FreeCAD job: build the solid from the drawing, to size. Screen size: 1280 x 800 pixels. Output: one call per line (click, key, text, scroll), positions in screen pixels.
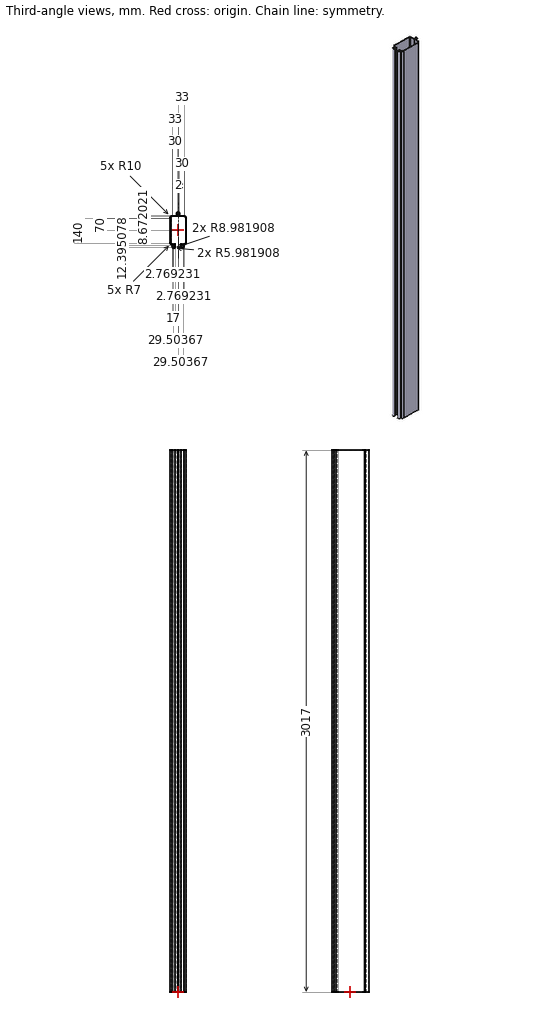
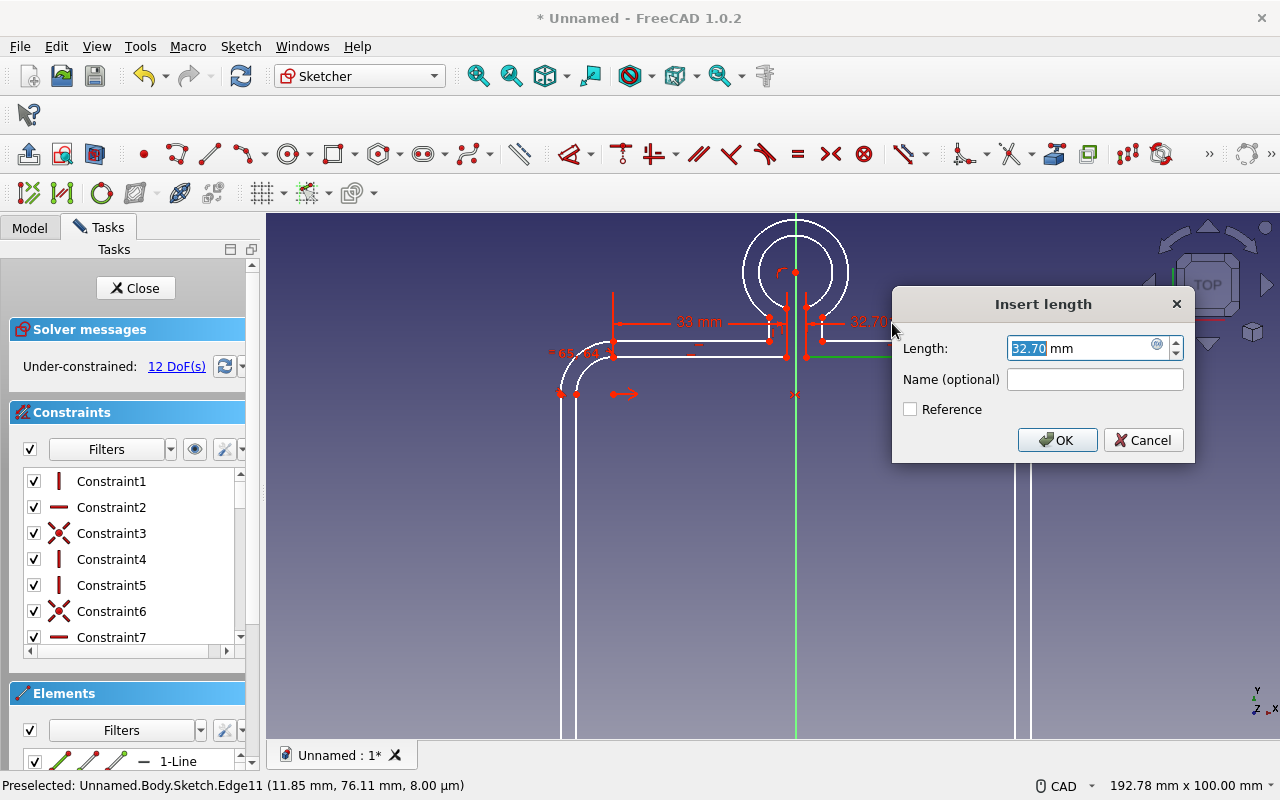
text(33)
key(Return)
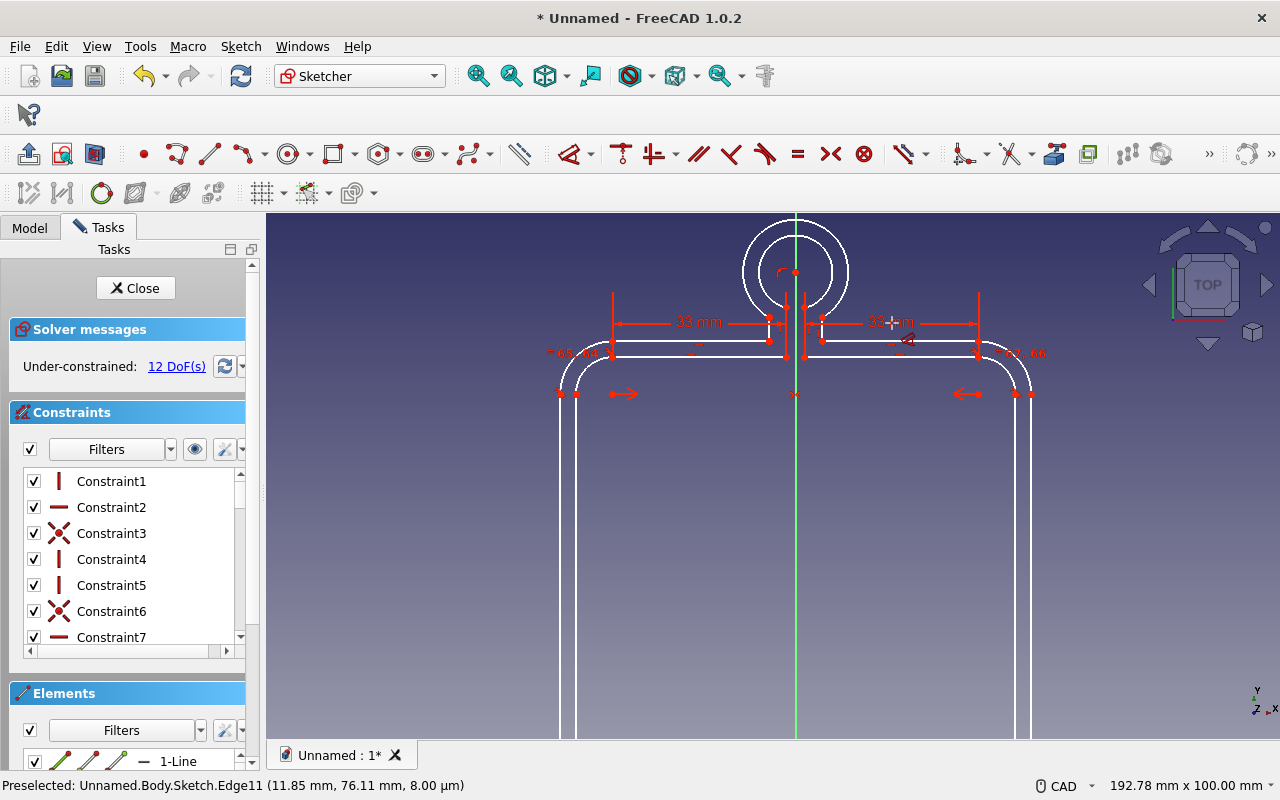
click(932, 341)
click(901, 375)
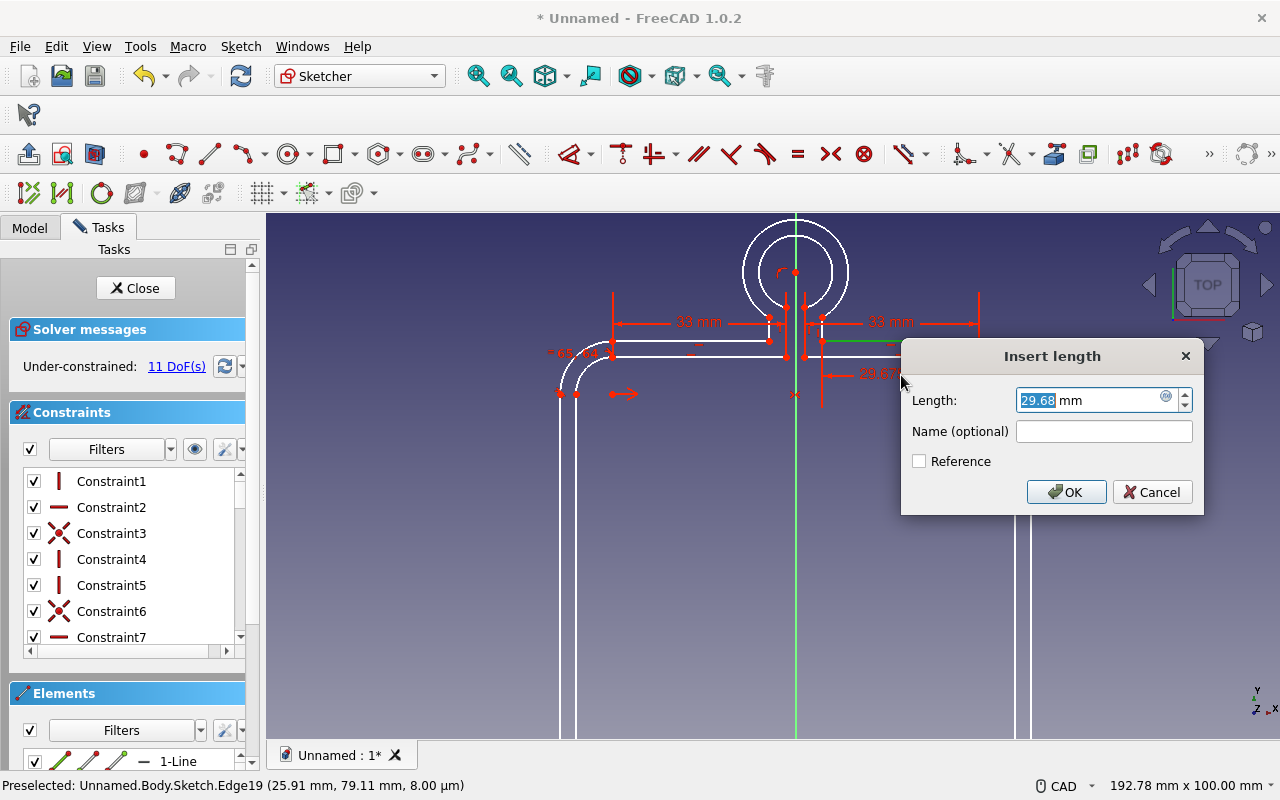
text(30)
key(Return)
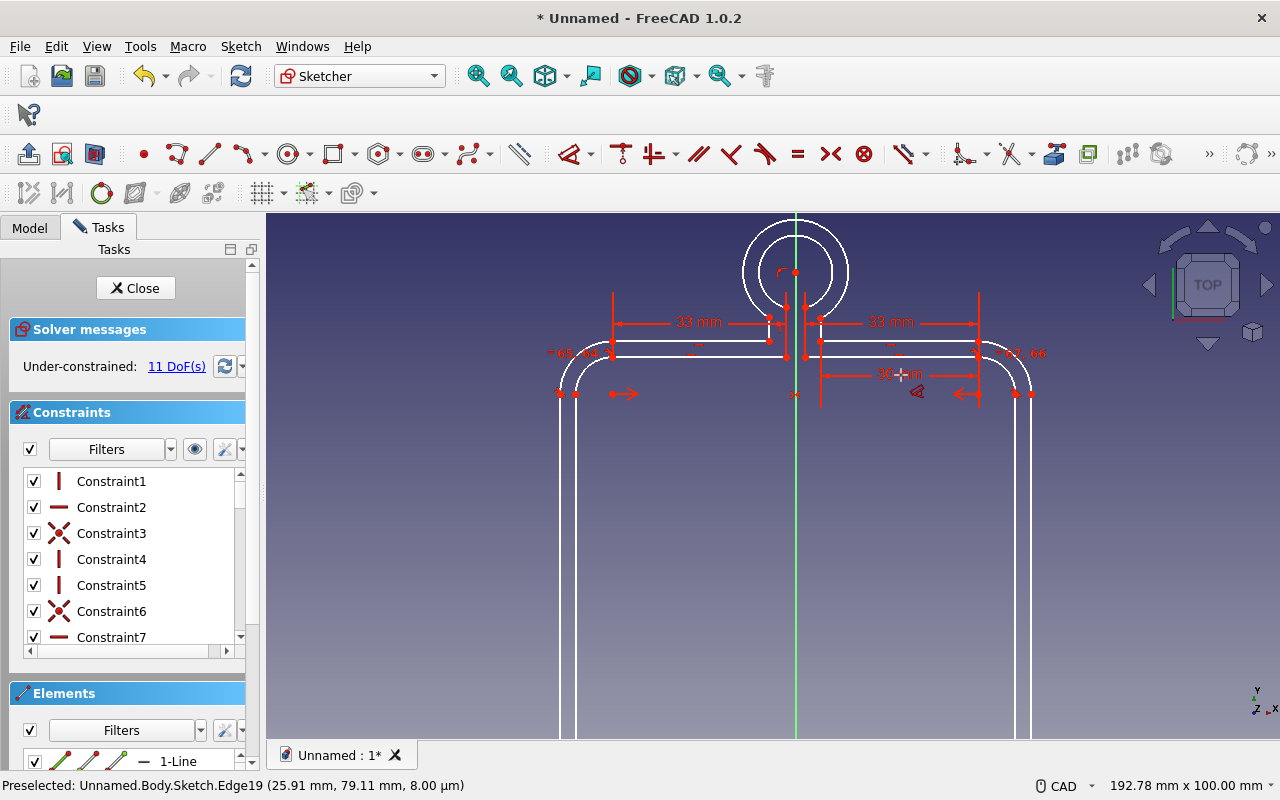
click(722, 341)
click(691, 375)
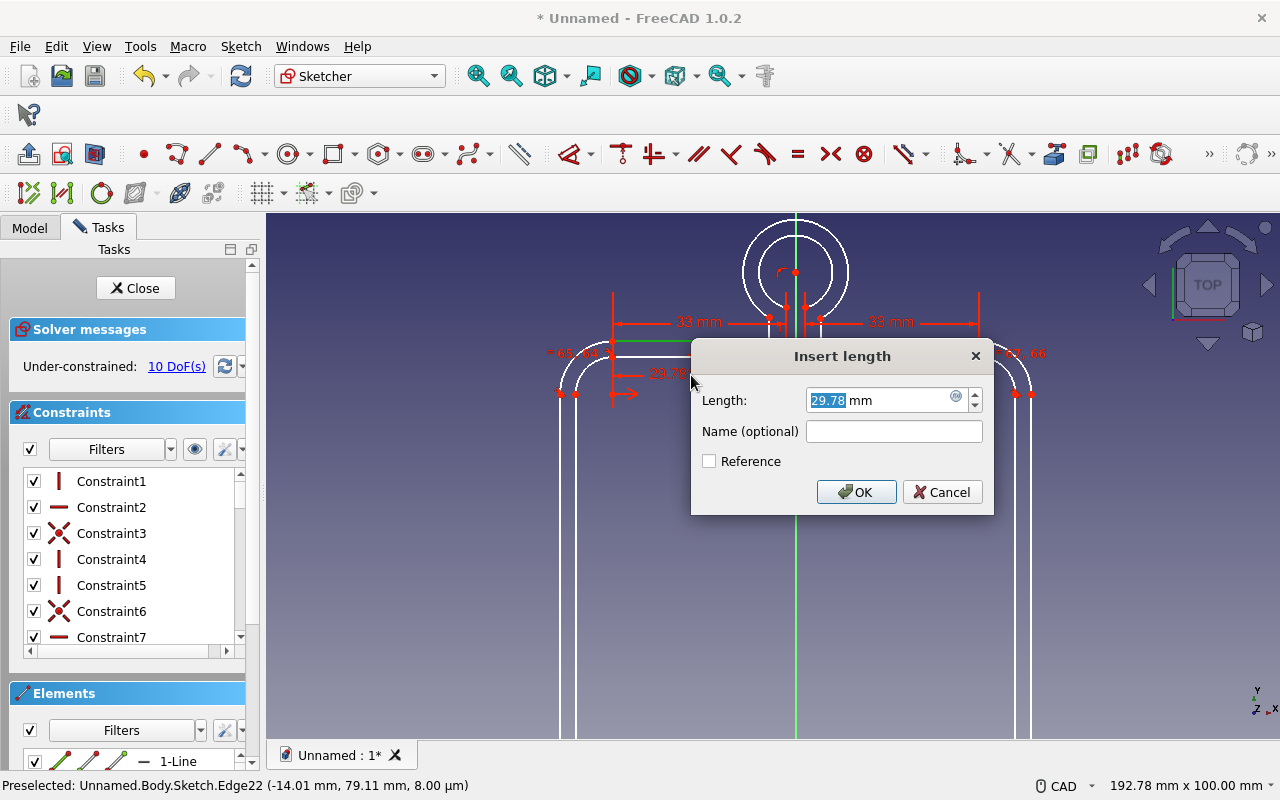
text(30)
key(Return)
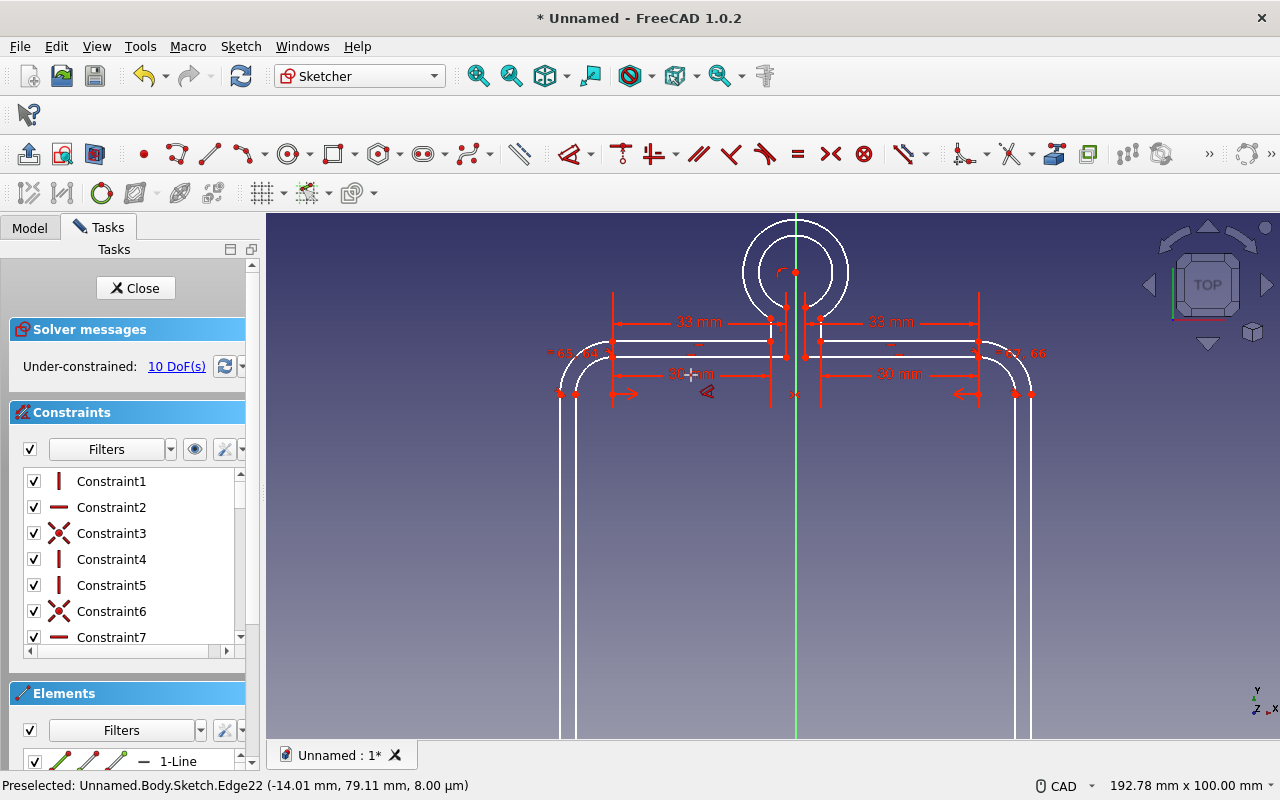
scroll(786, 357, up, 7)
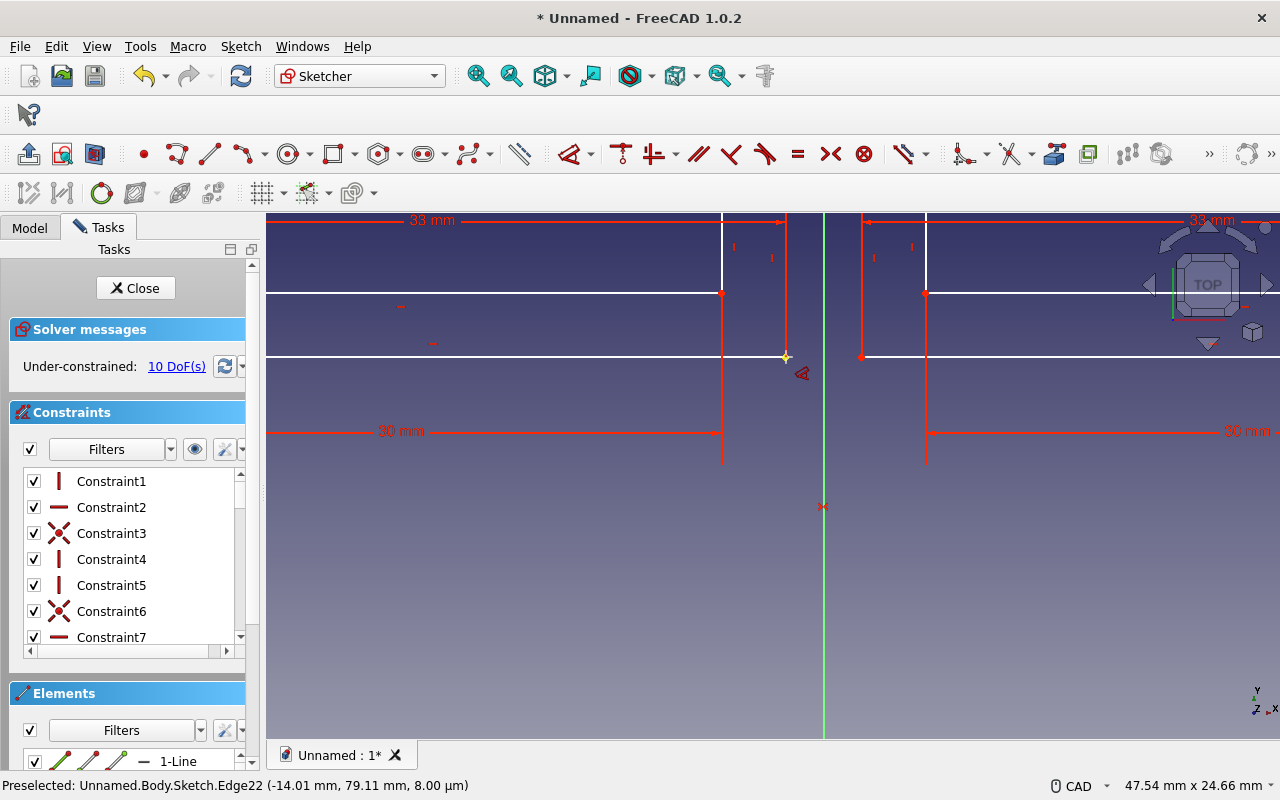
click(786, 357)
click(805, 323)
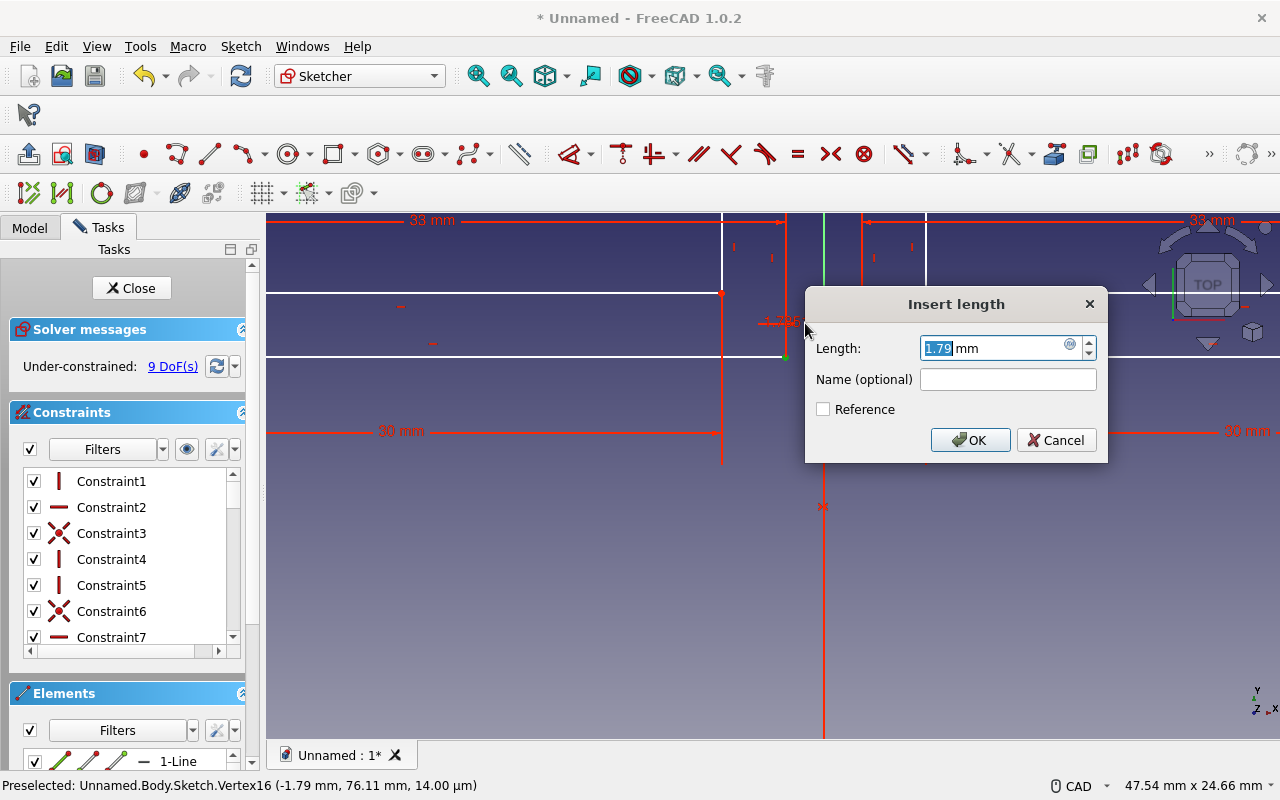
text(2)
key(Return)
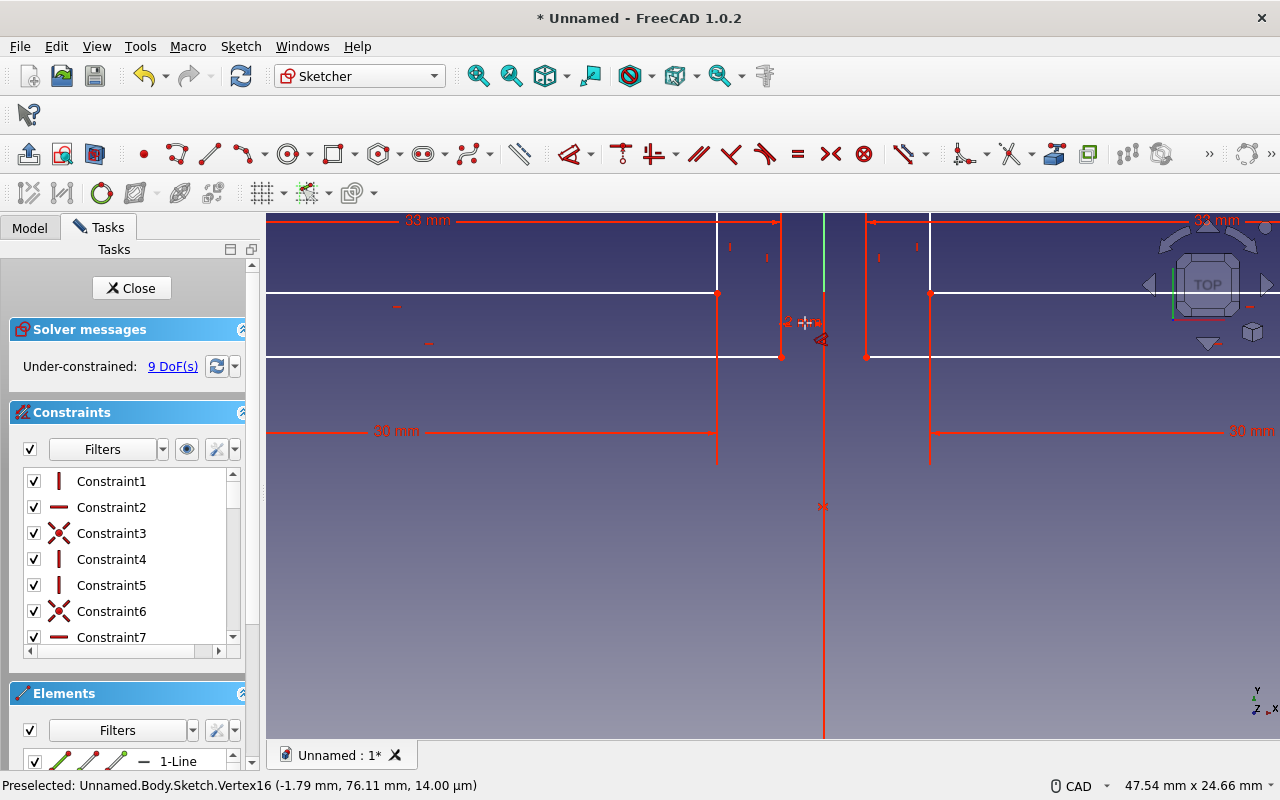
scroll(695, 356, down, 13)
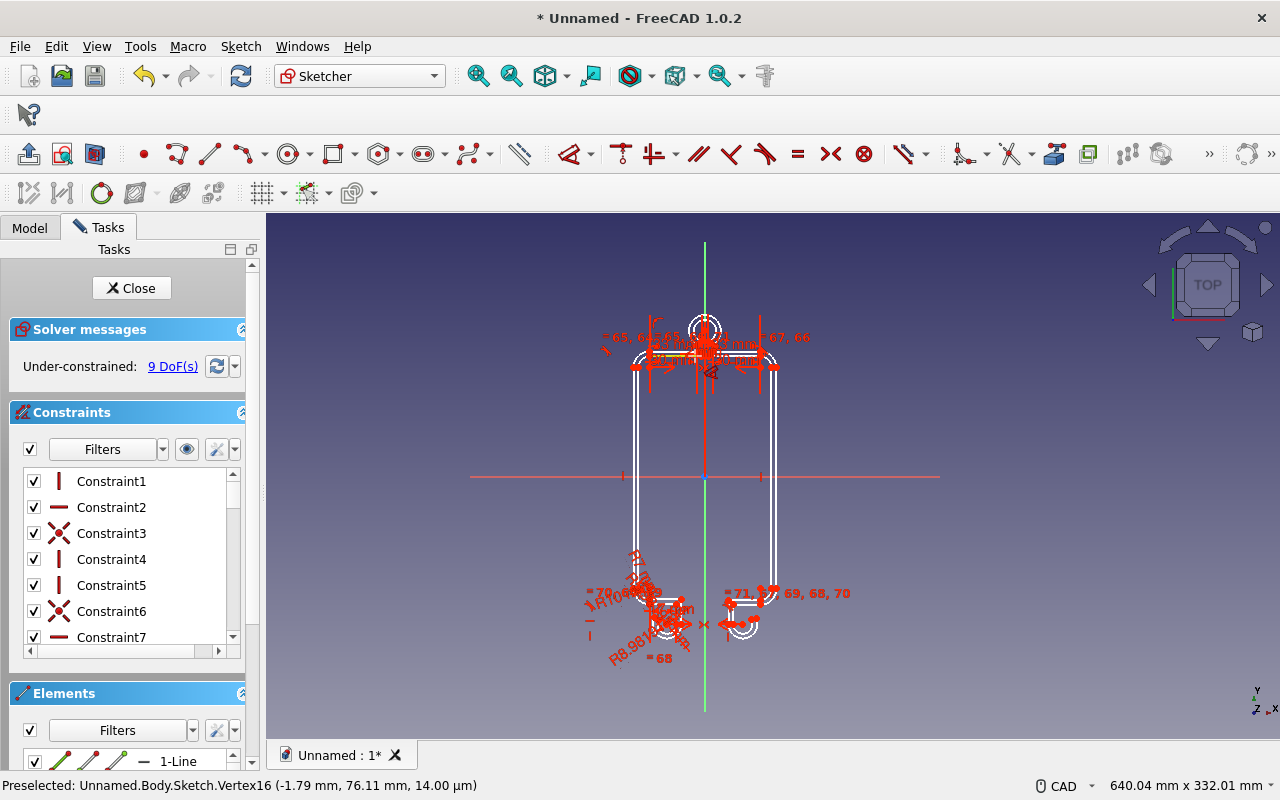
scroll(634, 434, up, 6)